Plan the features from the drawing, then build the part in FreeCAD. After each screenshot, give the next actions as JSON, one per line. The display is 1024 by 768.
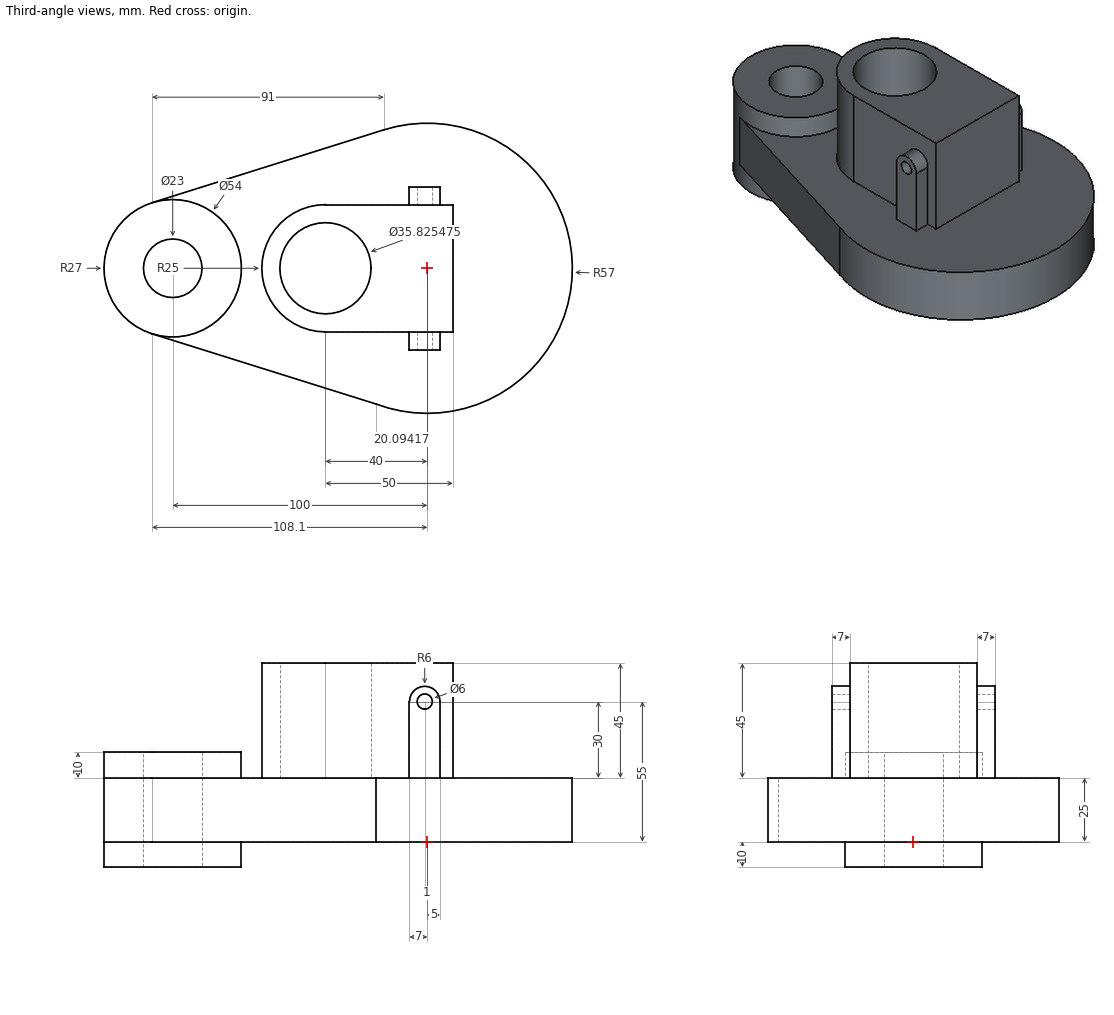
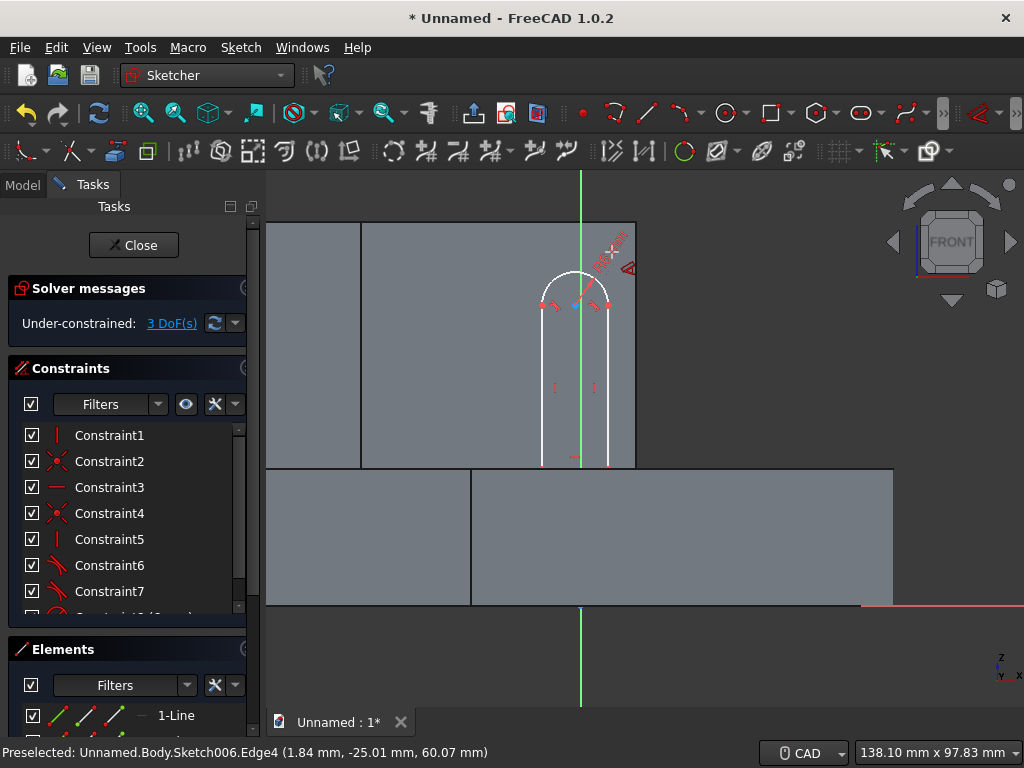
{"action": "left_click", "coordinate": [542, 355]}
{"action": "left_click", "coordinate": [508, 388]}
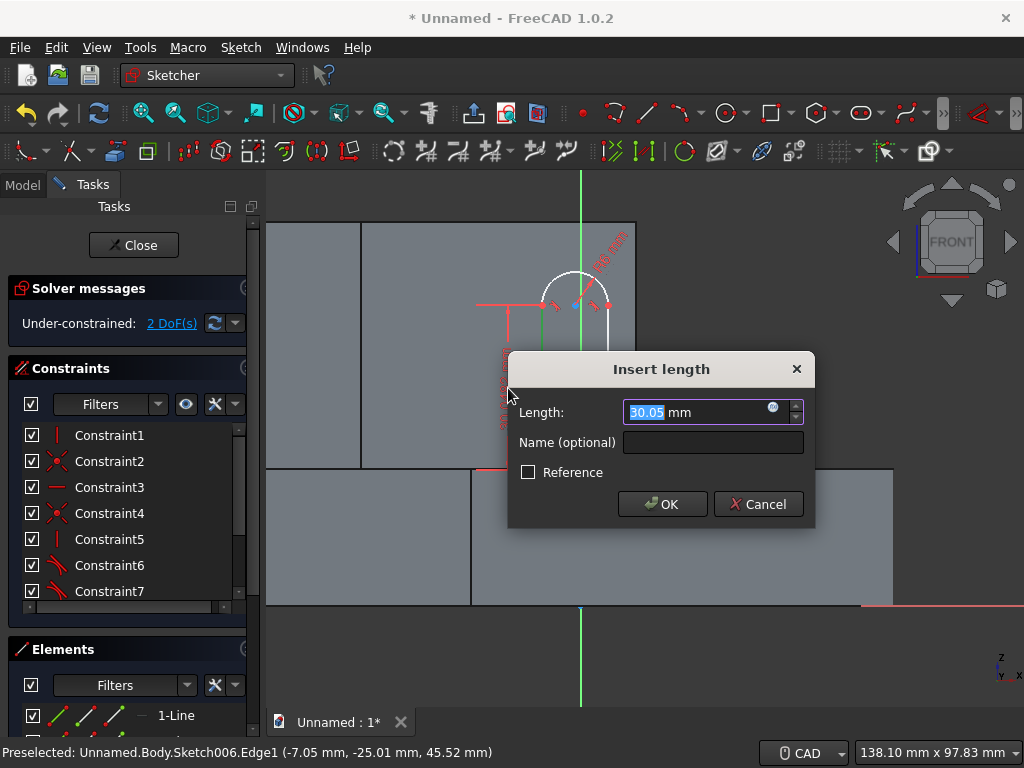
{"action": "type", "text": "30"}
{"action": "key", "text": "Return"}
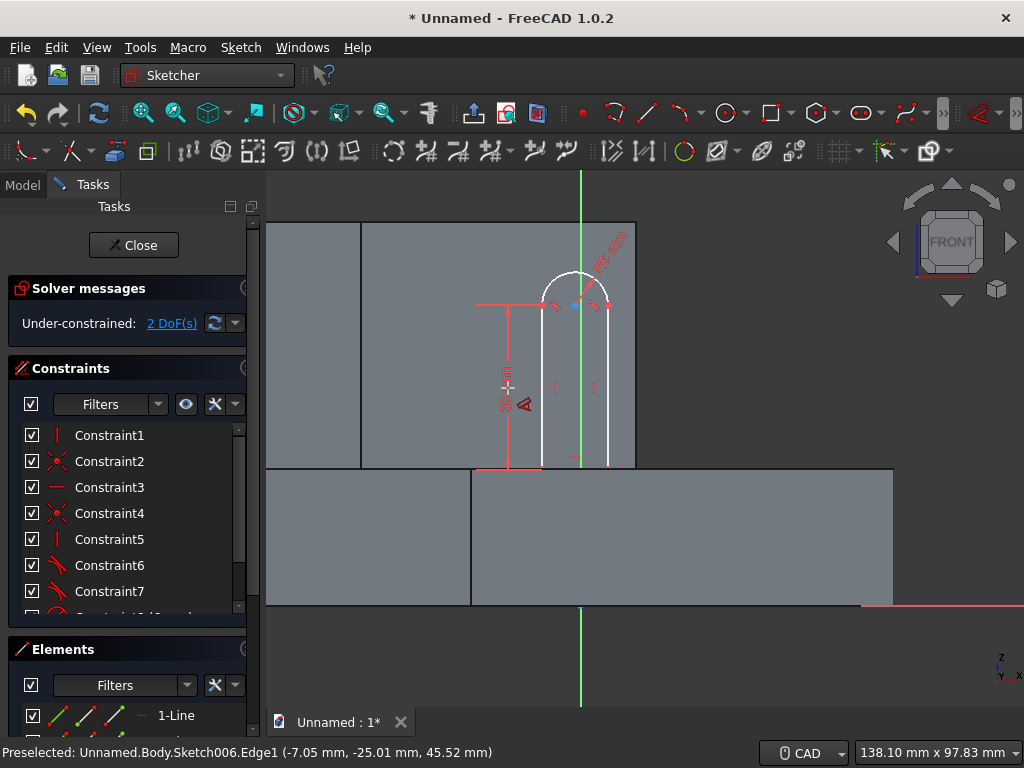
{"action": "left_click", "coordinate": [542, 305]}
{"action": "left_click", "coordinate": [561, 640]}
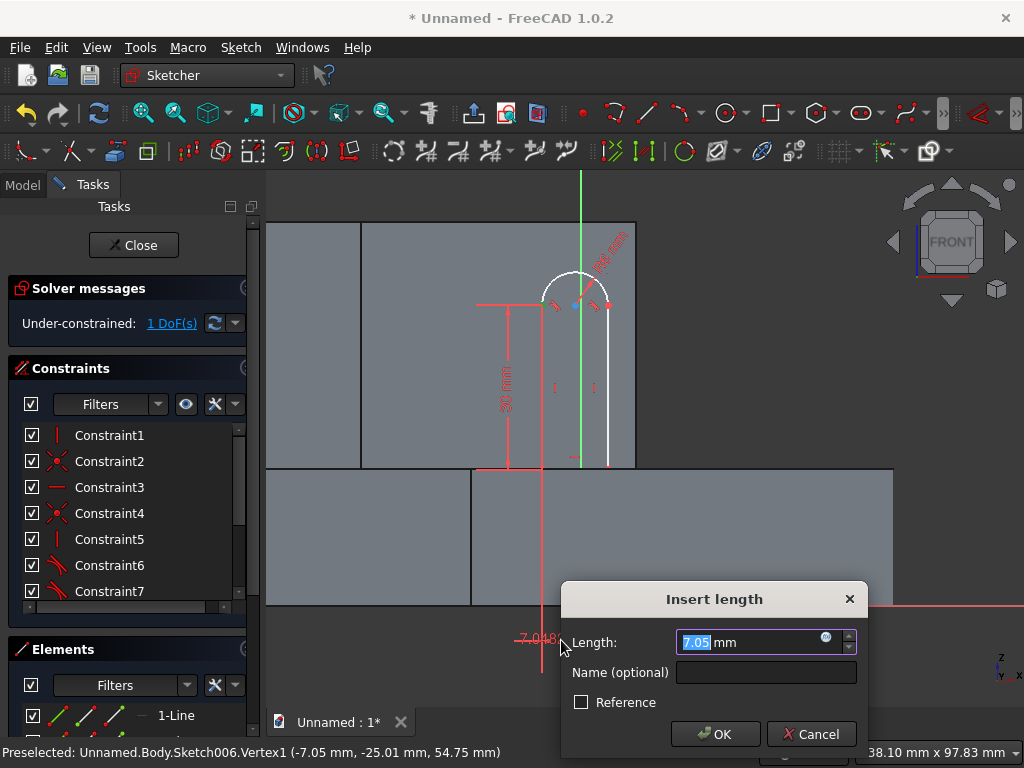
{"action": "type", "text": "7"}
{"action": "key", "text": "Return"}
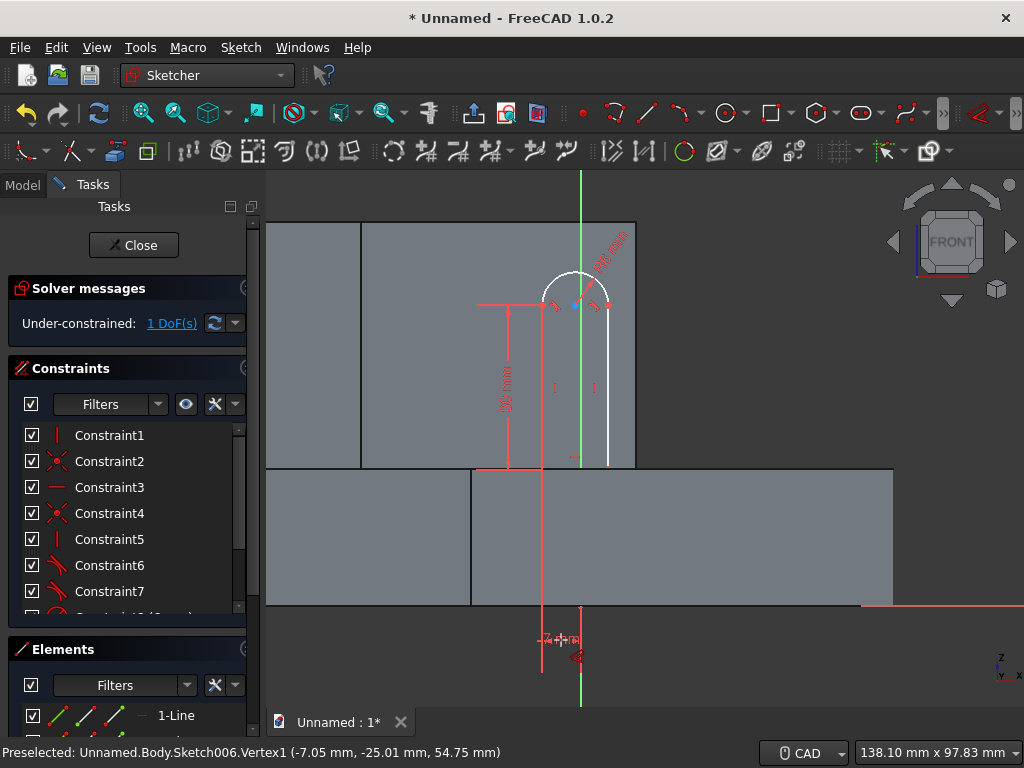
{"action": "left_click", "coordinate": [542, 305]}
{"action": "left_click", "coordinate": [508, 456]}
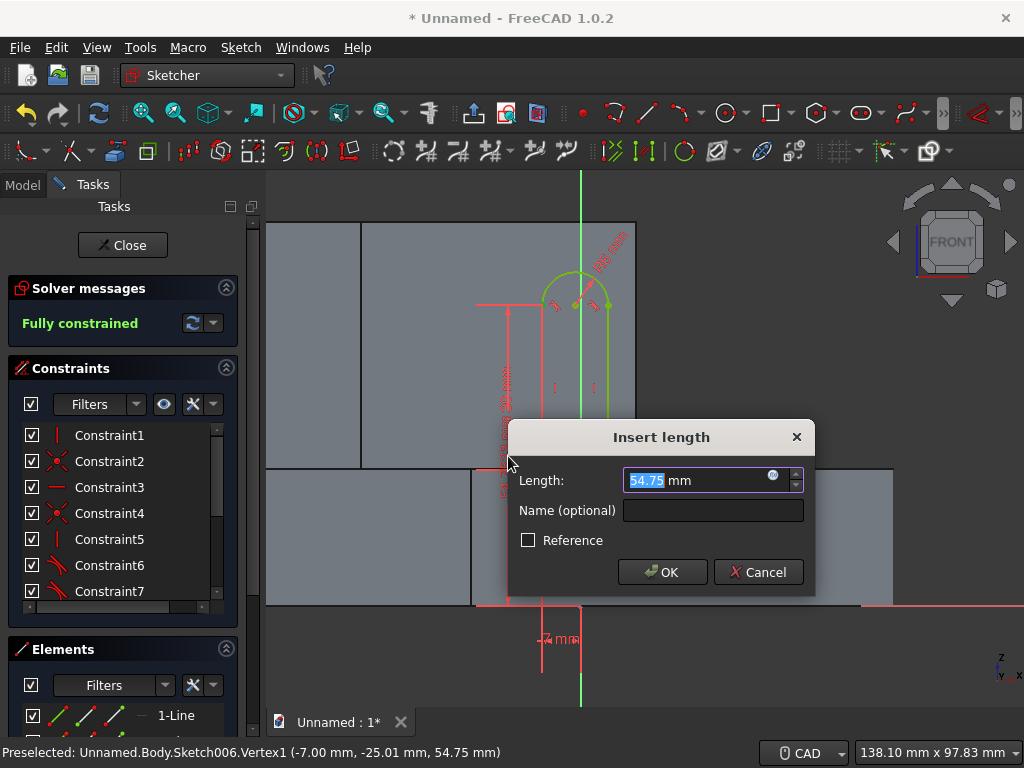
{"action": "type", "text": "55"}
{"action": "key", "text": "Return"}
{"action": "key", "text": "Escape"}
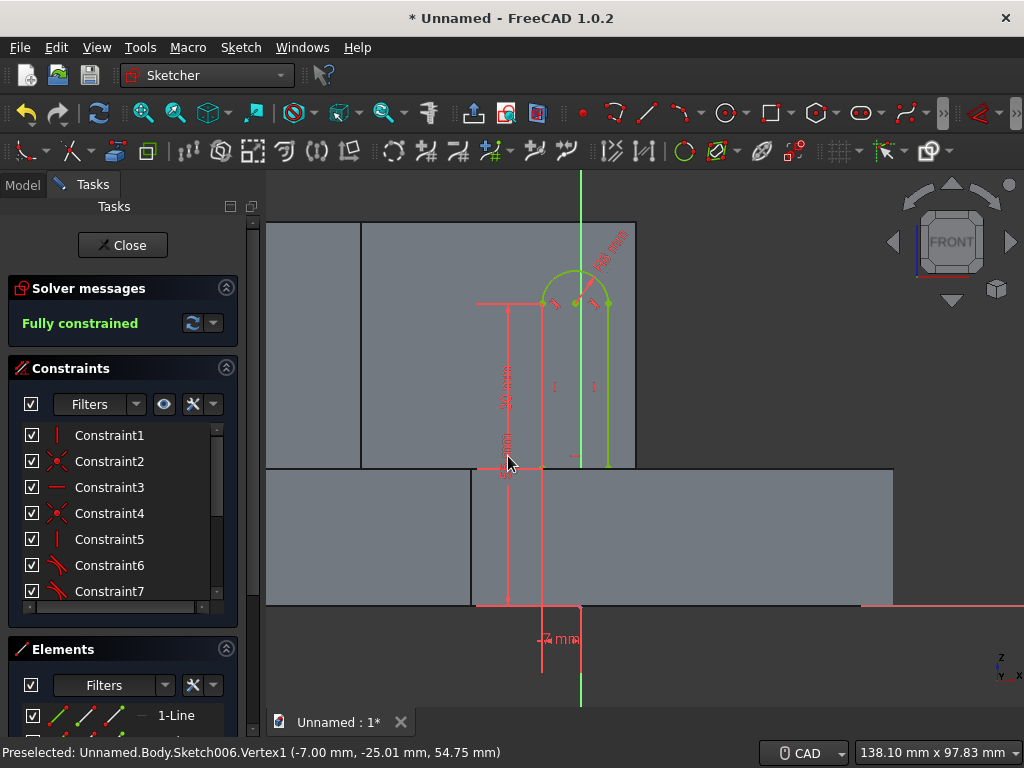
{"action": "left_click", "coordinate": [123, 245]}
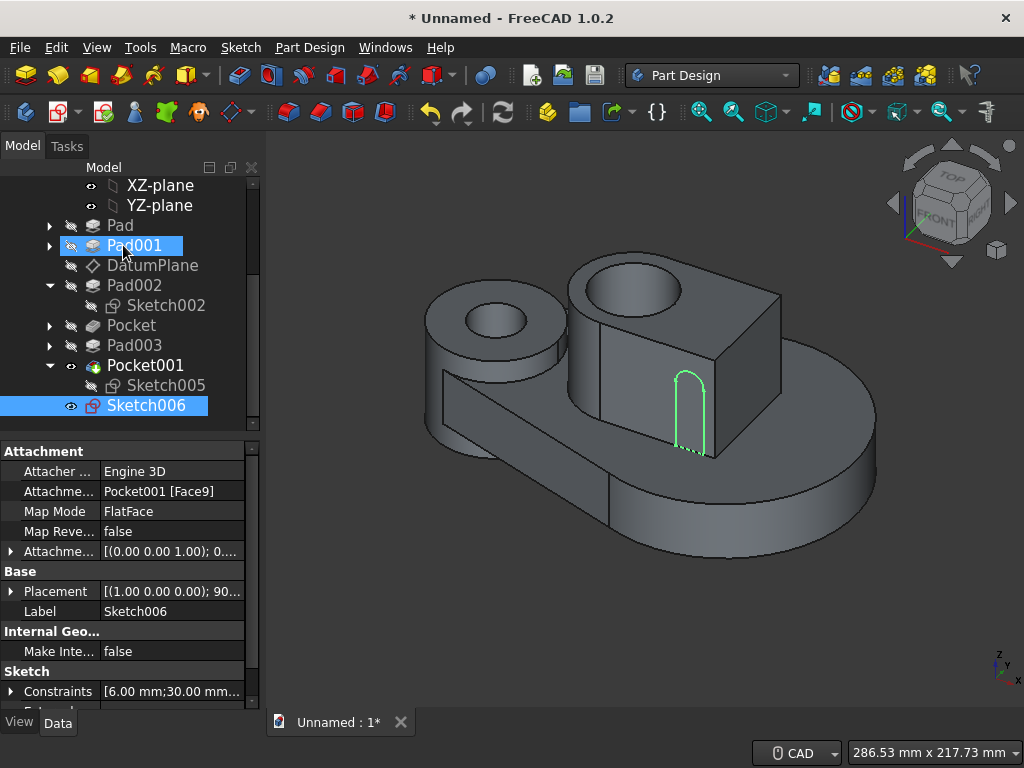
{"action": "left_click", "coordinate": [26, 76]}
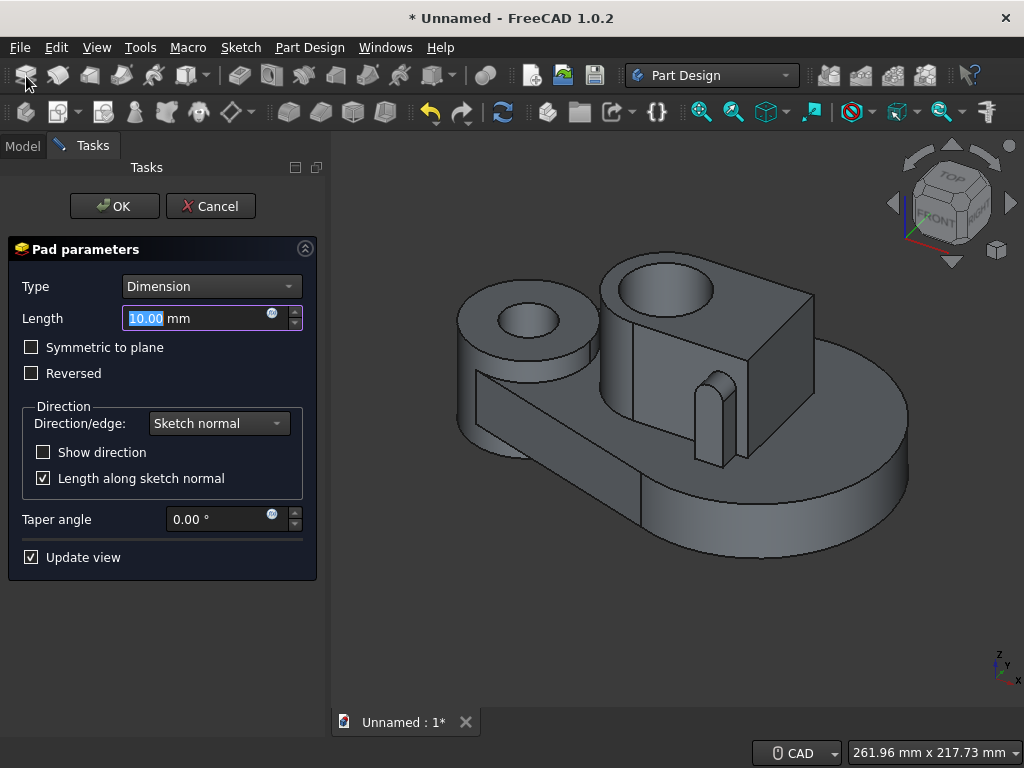
{"action": "type", "text": "7"}
{"action": "key", "text": "Tab"}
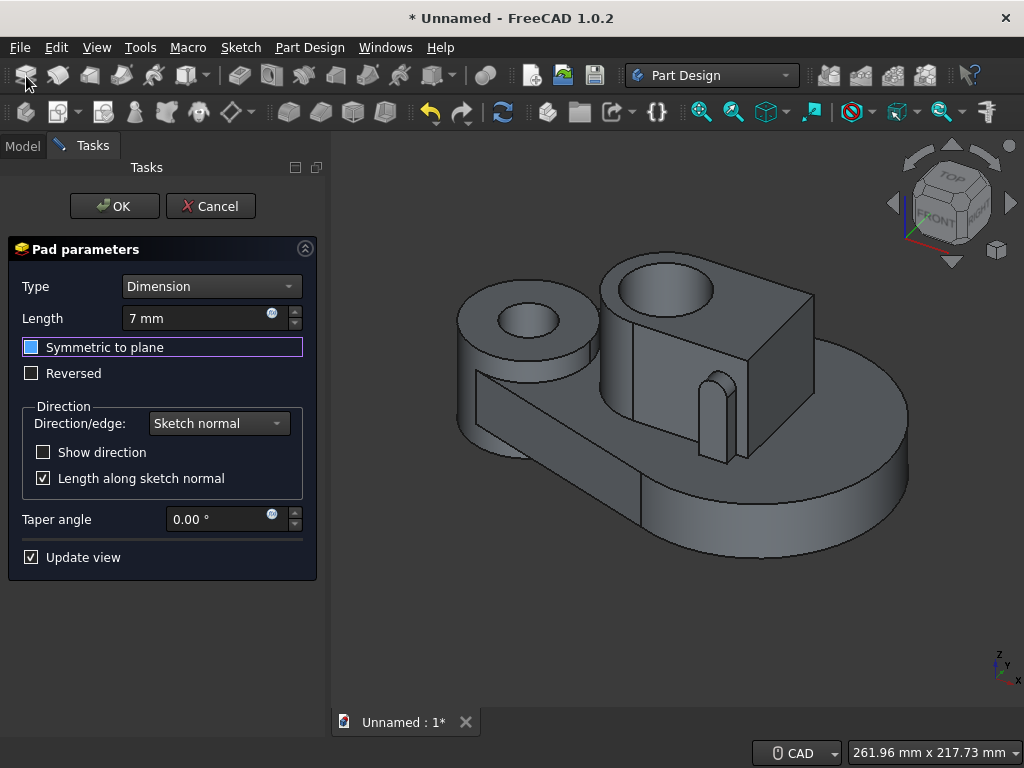
{"action": "left_click", "coordinate": [115, 206]}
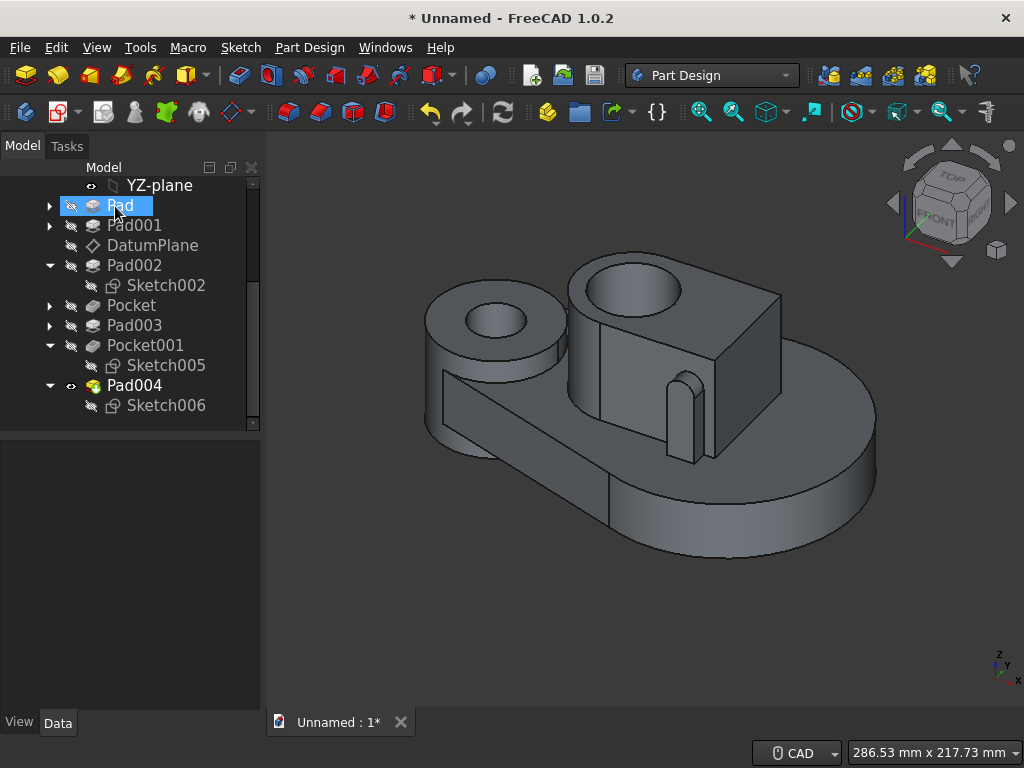
{"action": "scroll", "coordinate": [160, 301], "scroll_direction": "down", "scroll_amount": 3}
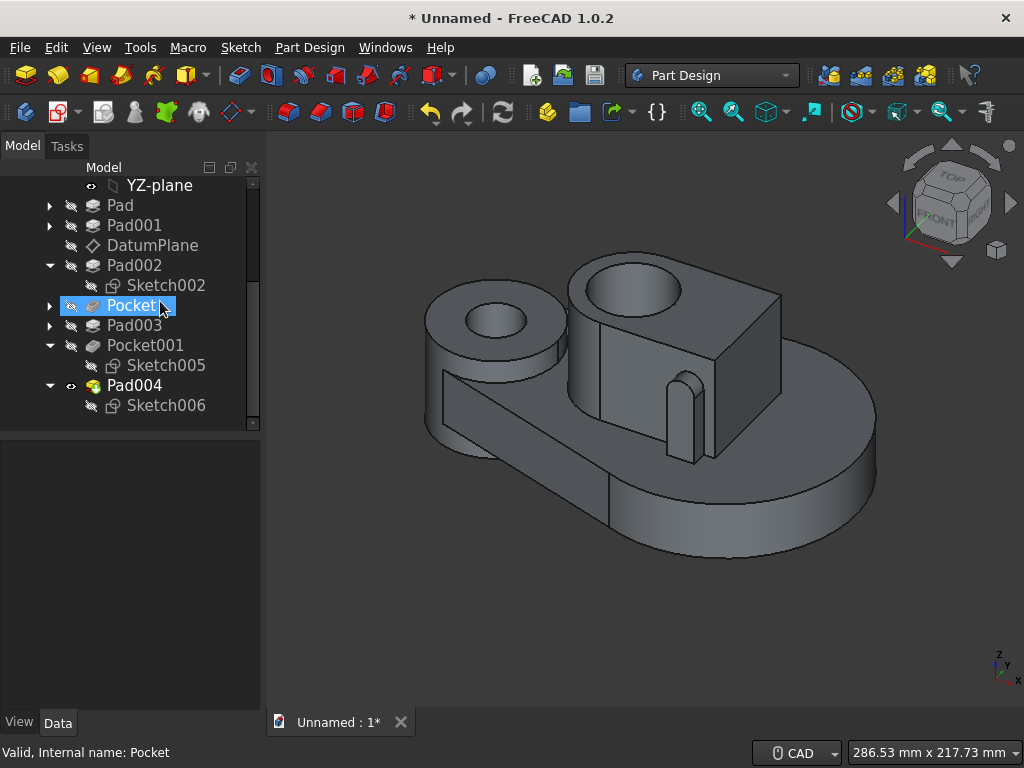
{"action": "scroll", "coordinate": [160, 301], "scroll_direction": "up", "scroll_amount": 15}